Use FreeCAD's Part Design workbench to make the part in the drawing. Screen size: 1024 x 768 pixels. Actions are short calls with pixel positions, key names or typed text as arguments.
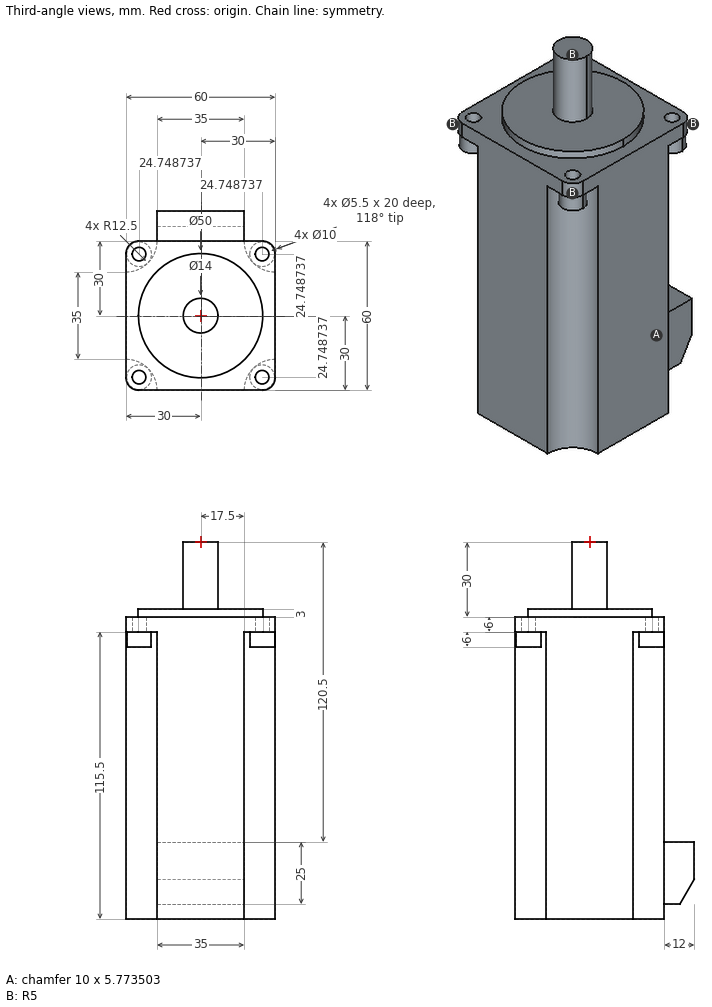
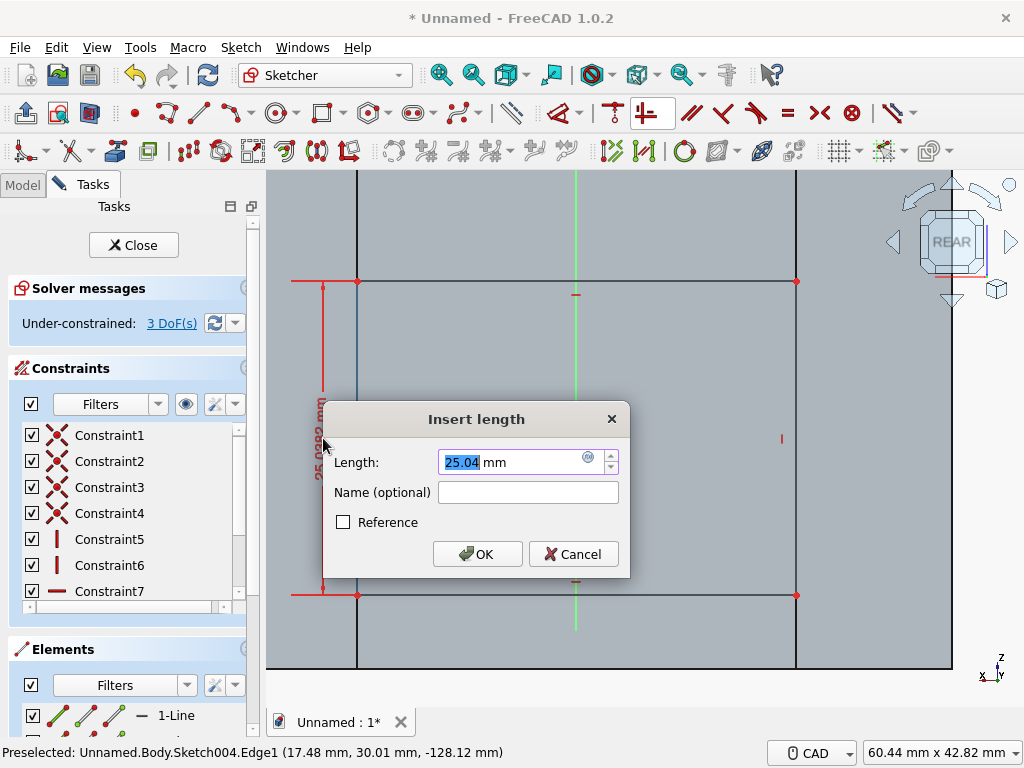
text(25)
key(Return)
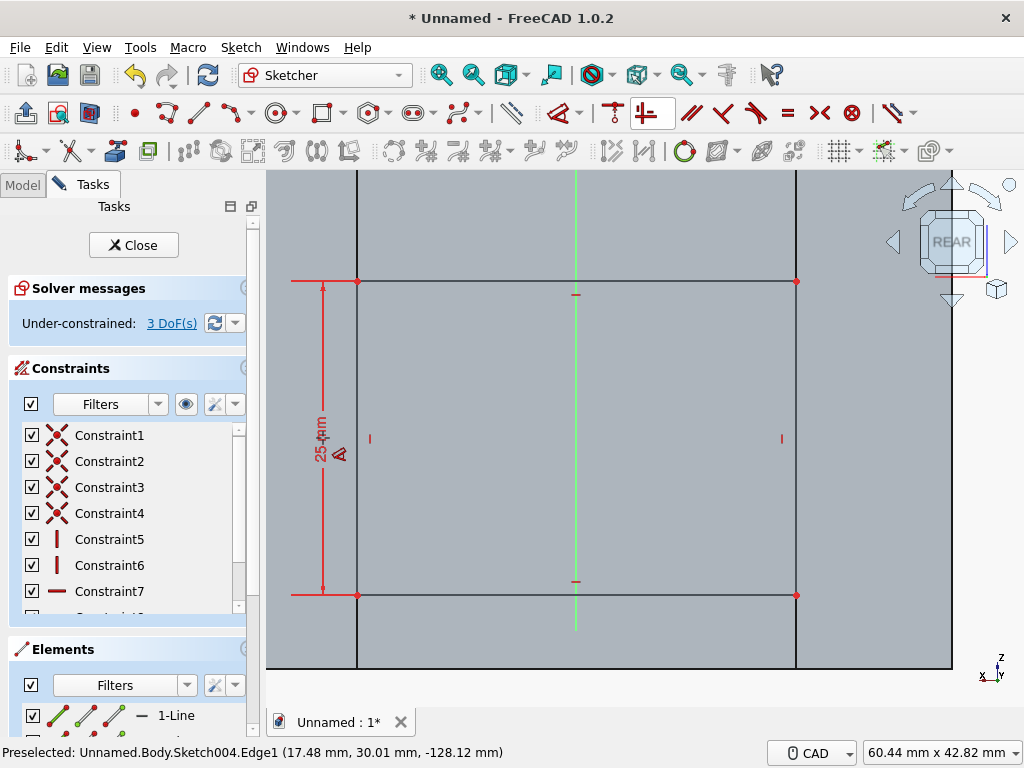
click(489, 595)
click(476, 629)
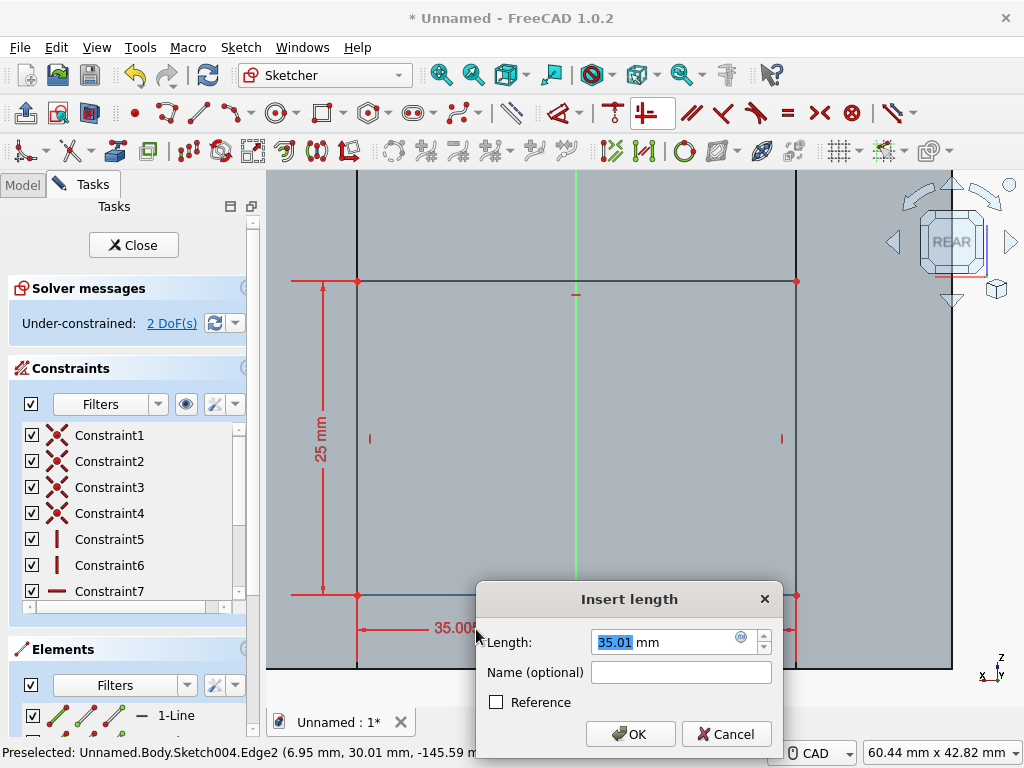
text(35)
key(Return)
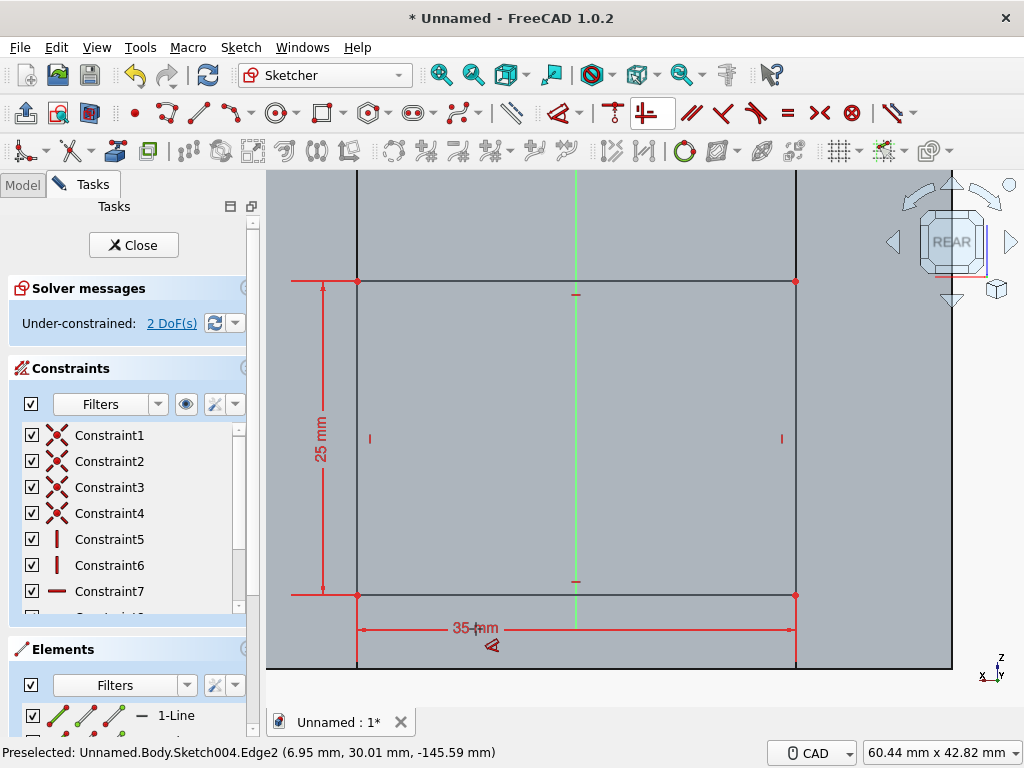
click(357, 281)
click(467, 315)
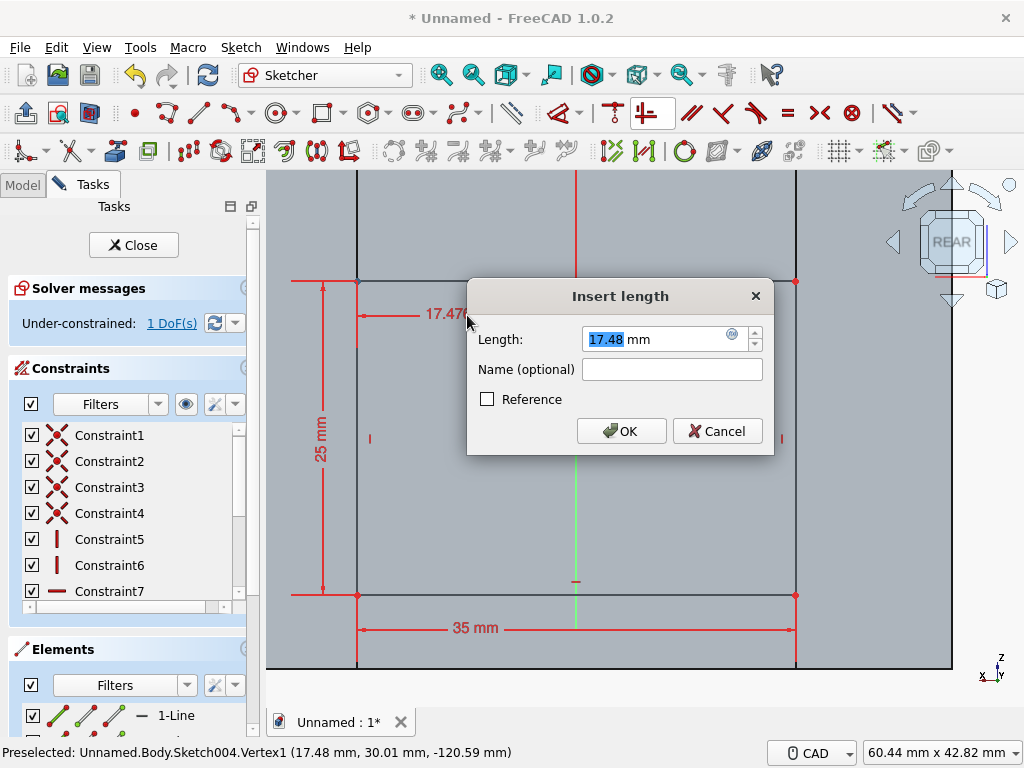
text(17.5)
key(Return)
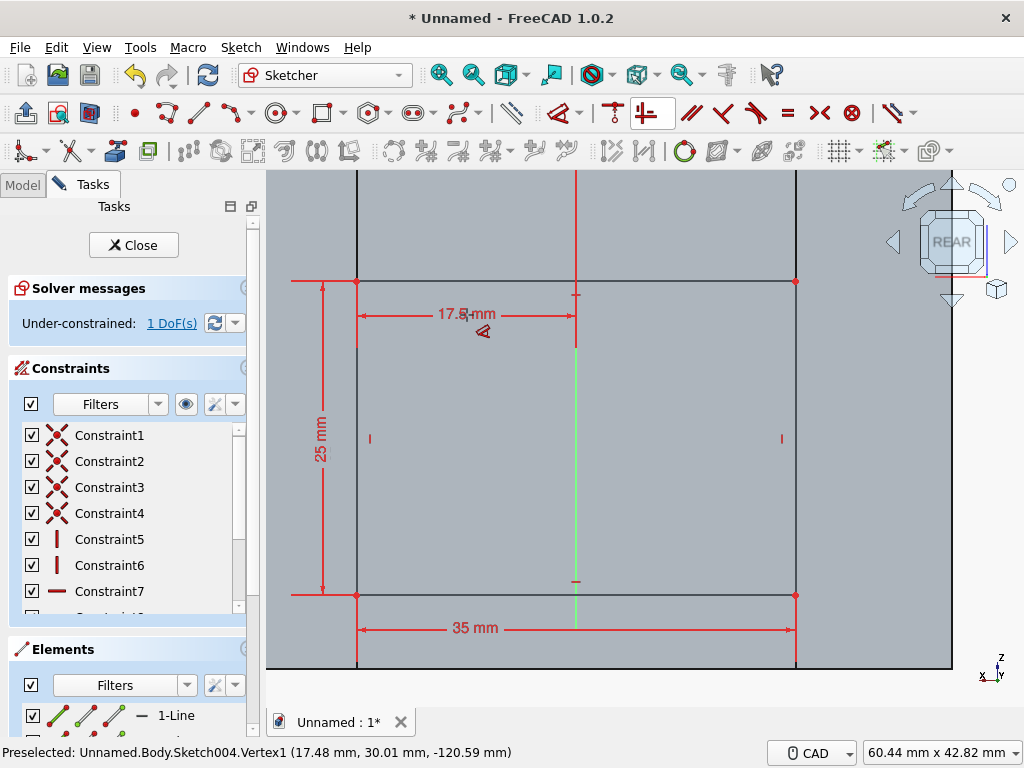
click(357, 281)
click(323, 240)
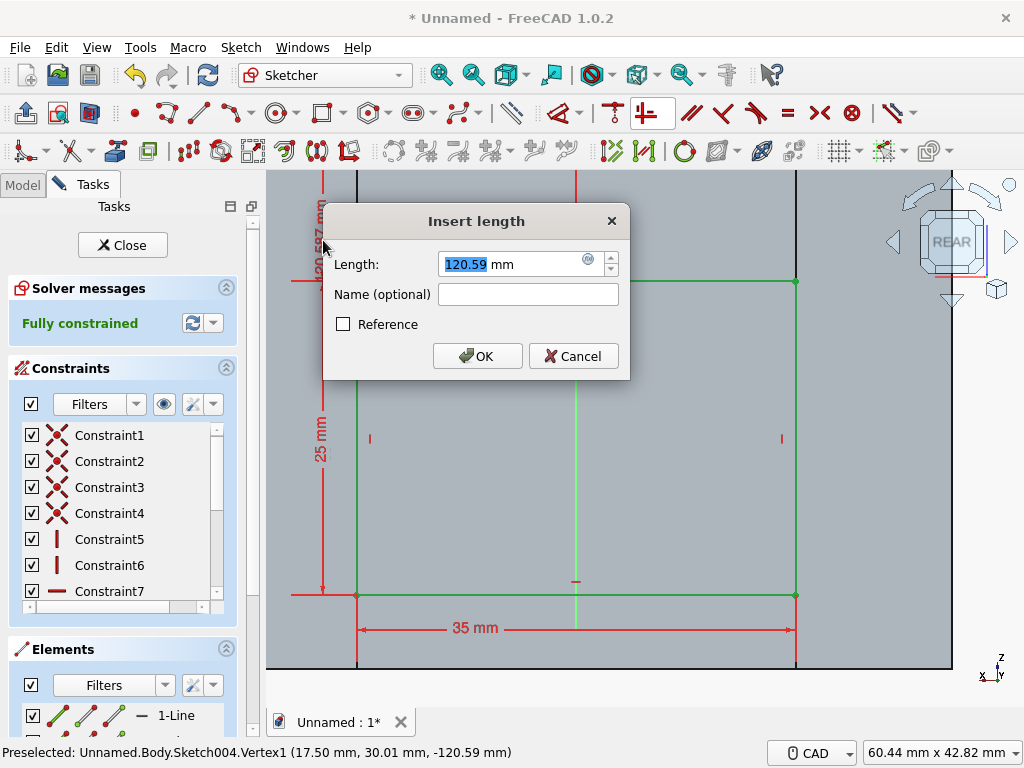
text(120.5)
key(Return)
key(Escape)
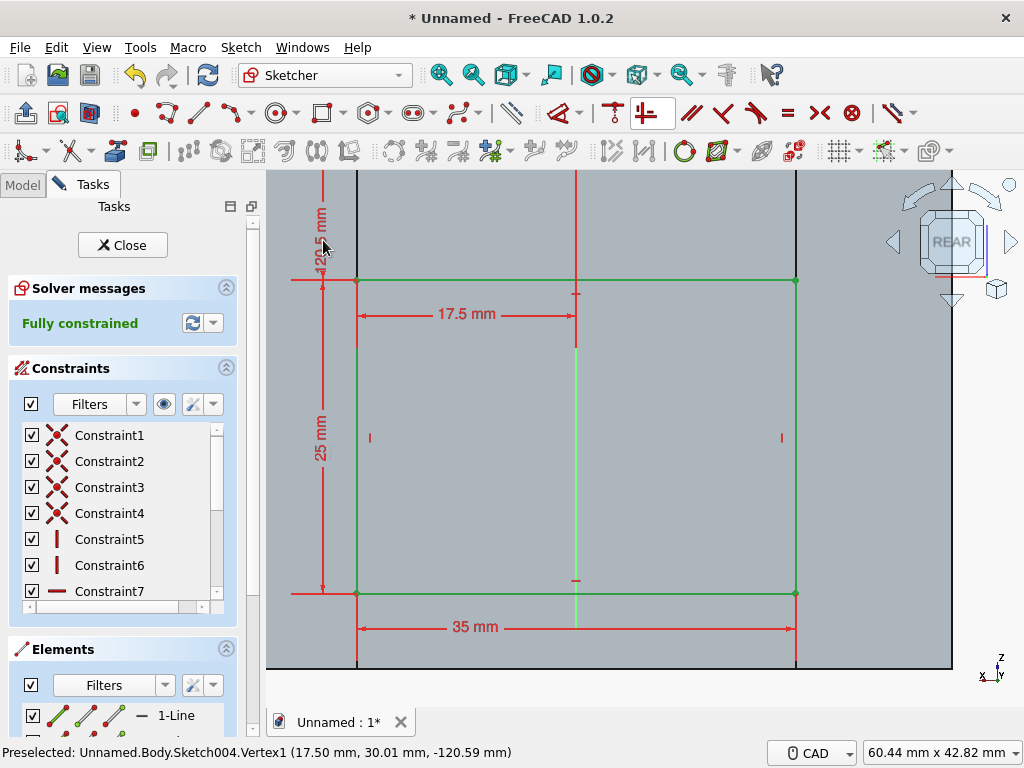
click(123, 245)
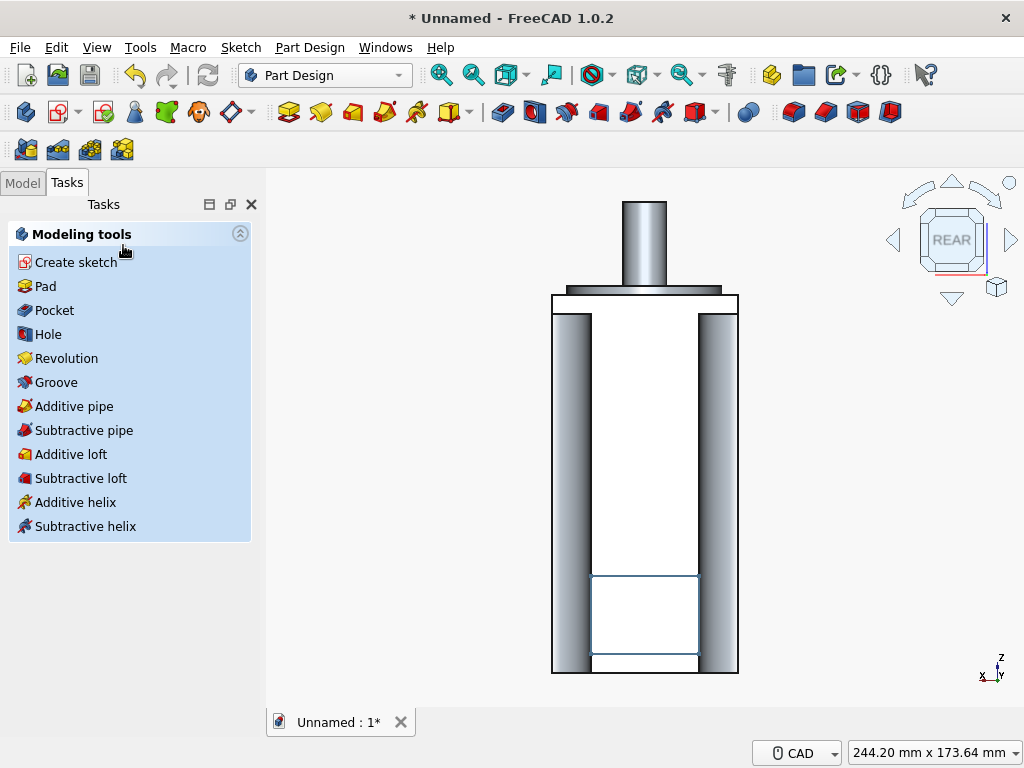
click(290, 112)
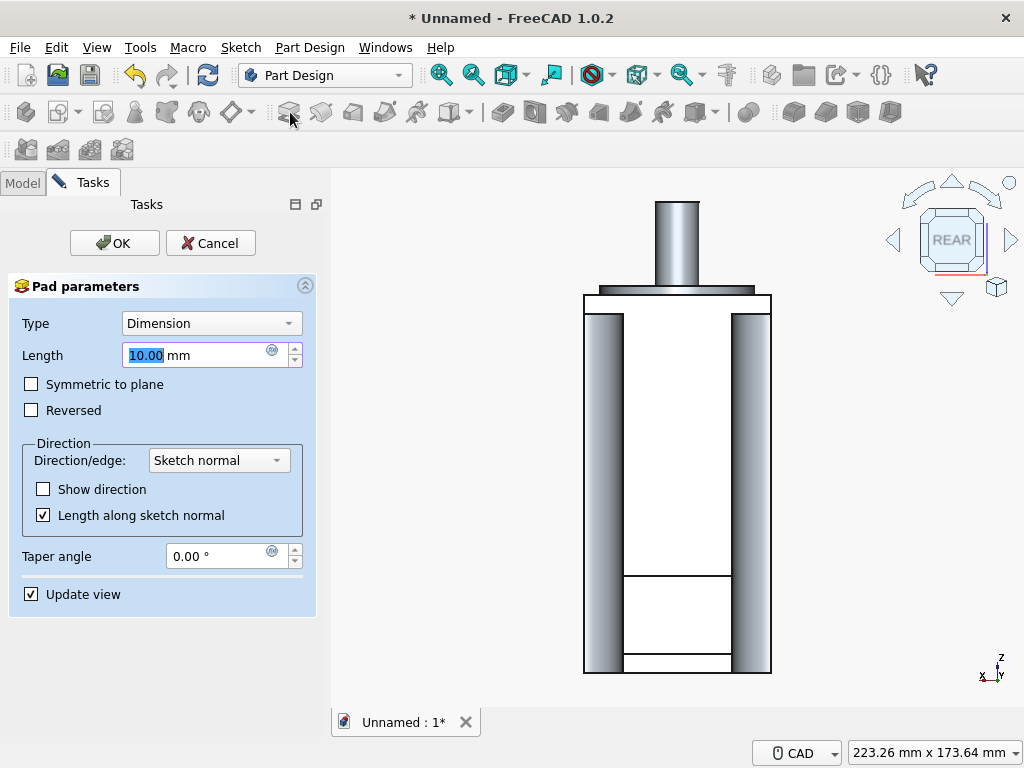
text(12)
key(Tab)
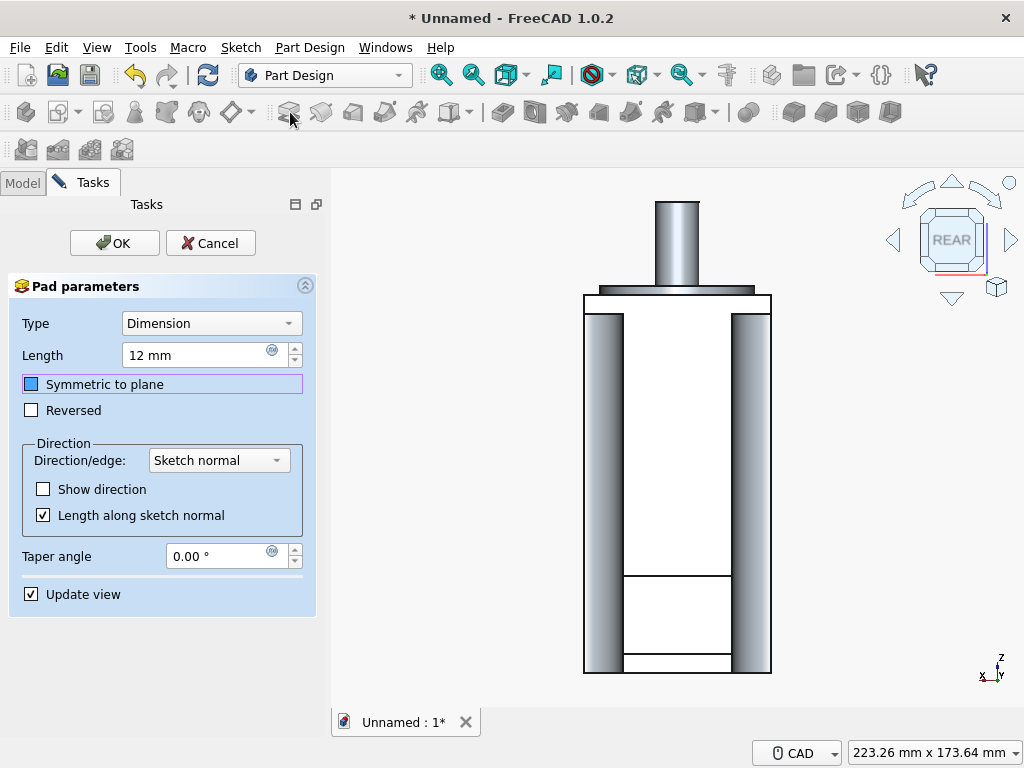
click(115, 243)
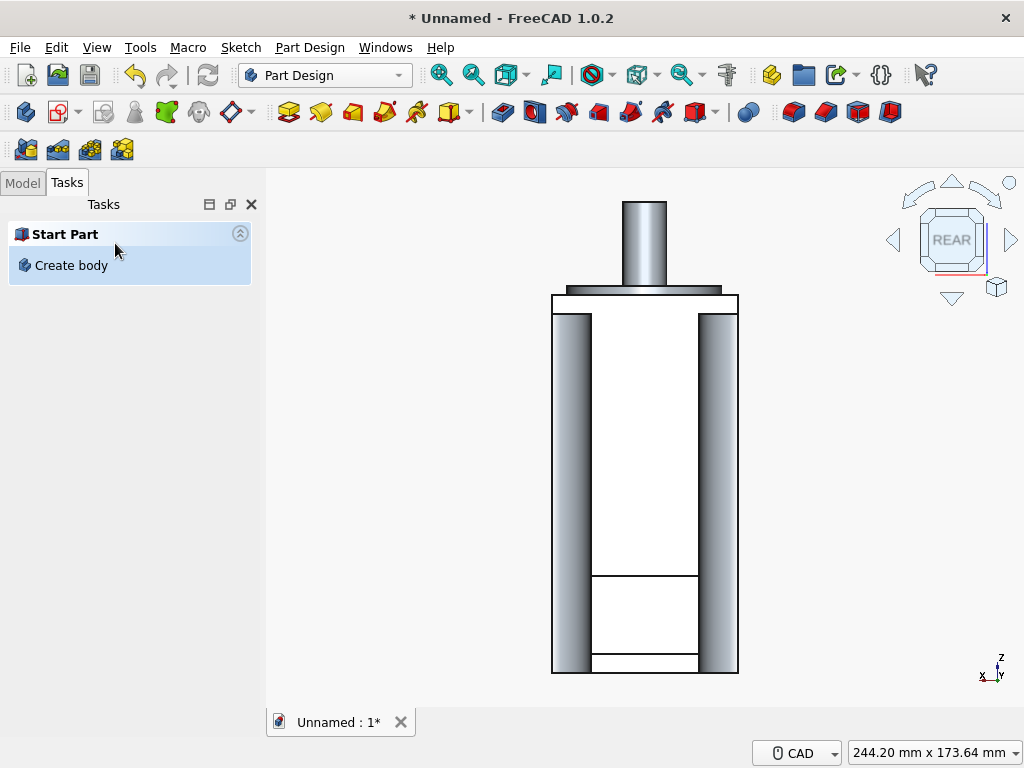
click(645, 653)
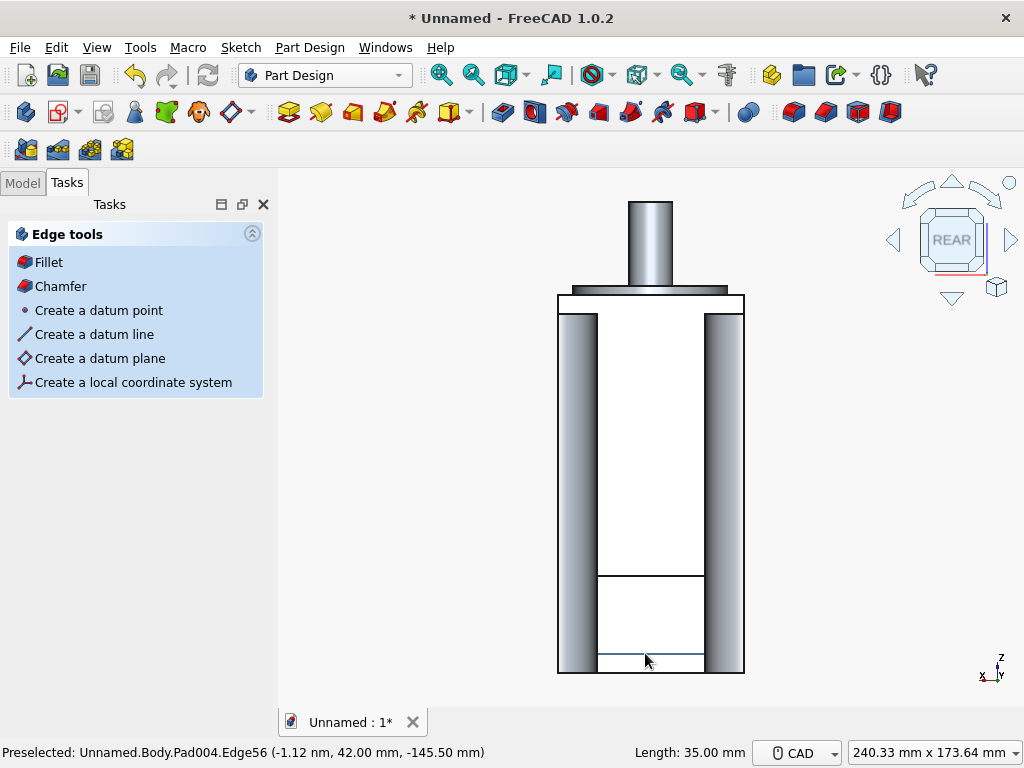
click(826, 112)